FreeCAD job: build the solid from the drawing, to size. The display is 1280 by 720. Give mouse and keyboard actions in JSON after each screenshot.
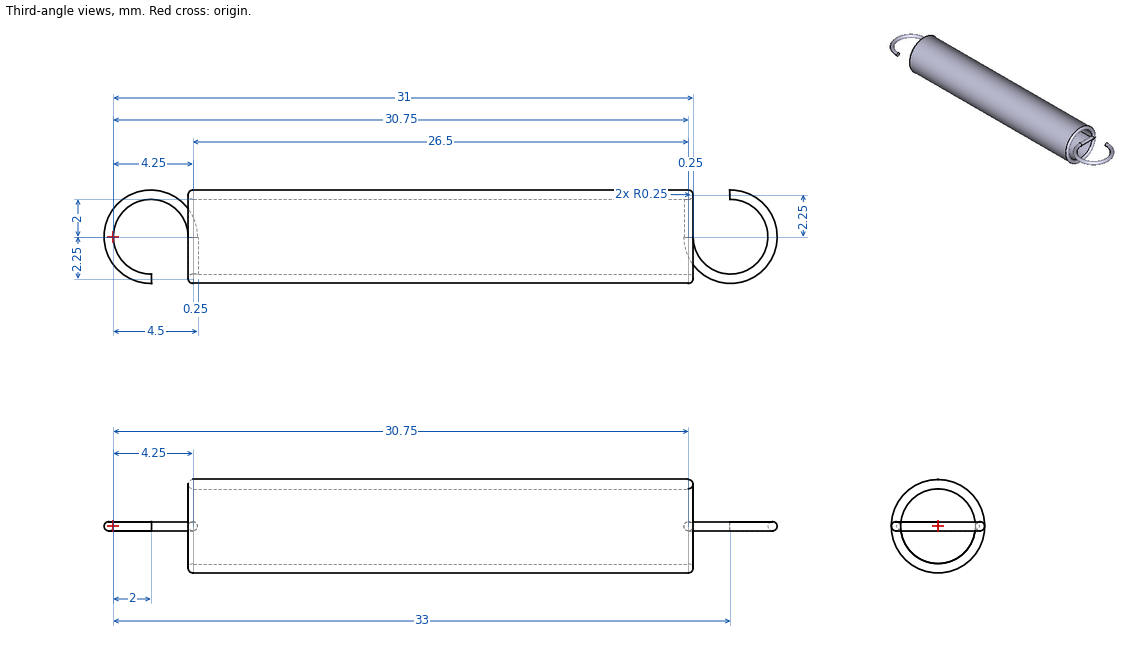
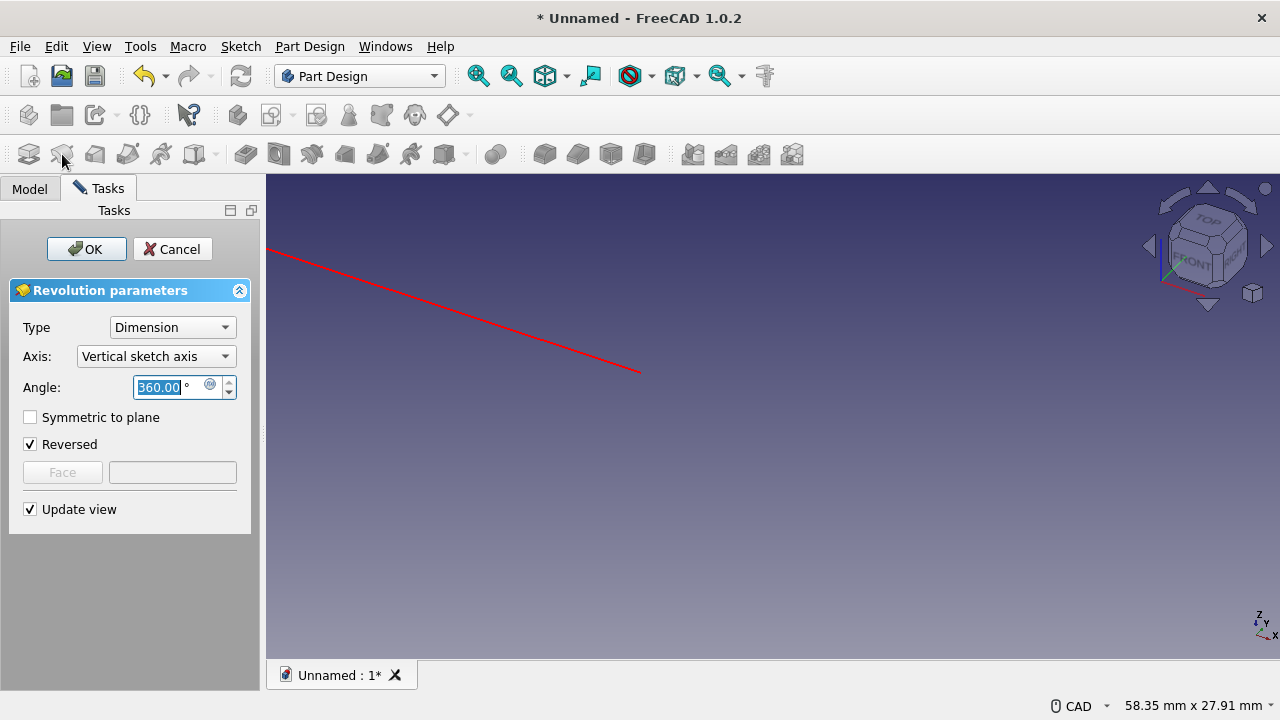
{"action": "left_click", "coordinate": [157, 356]}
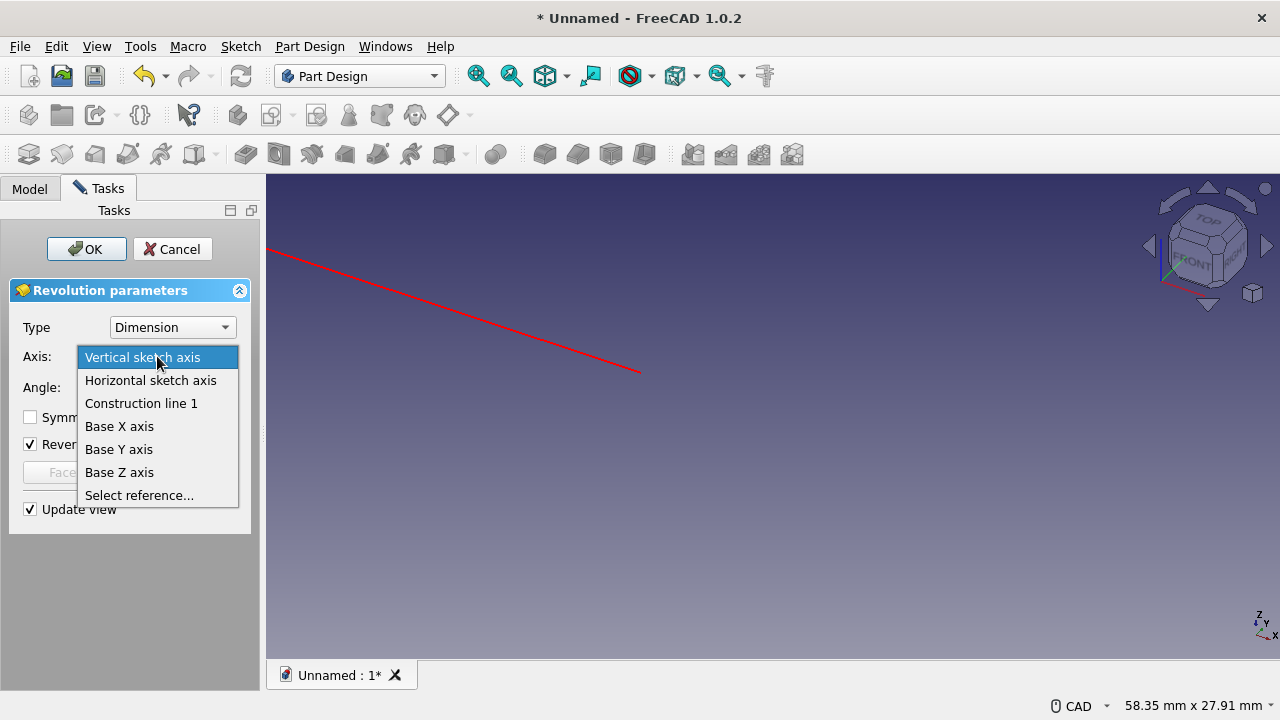
{"action": "left_click", "coordinate": [156, 404]}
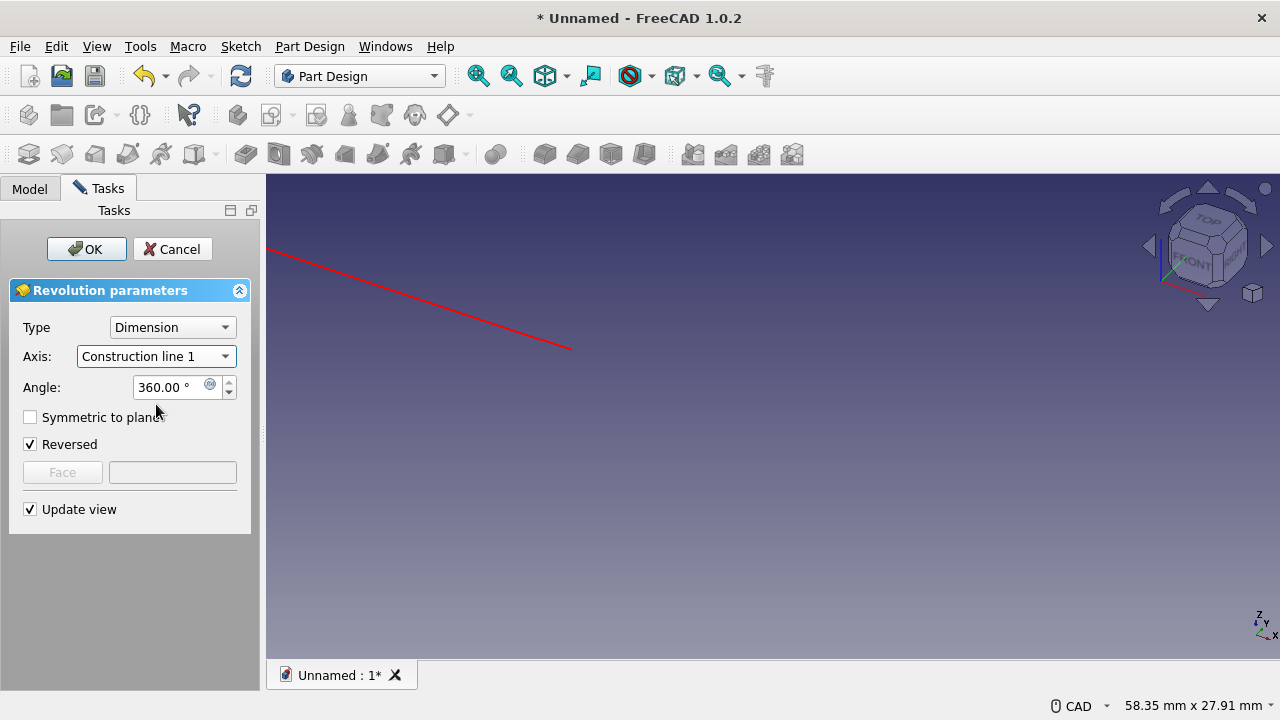
{"action": "left_click", "coordinate": [87, 249]}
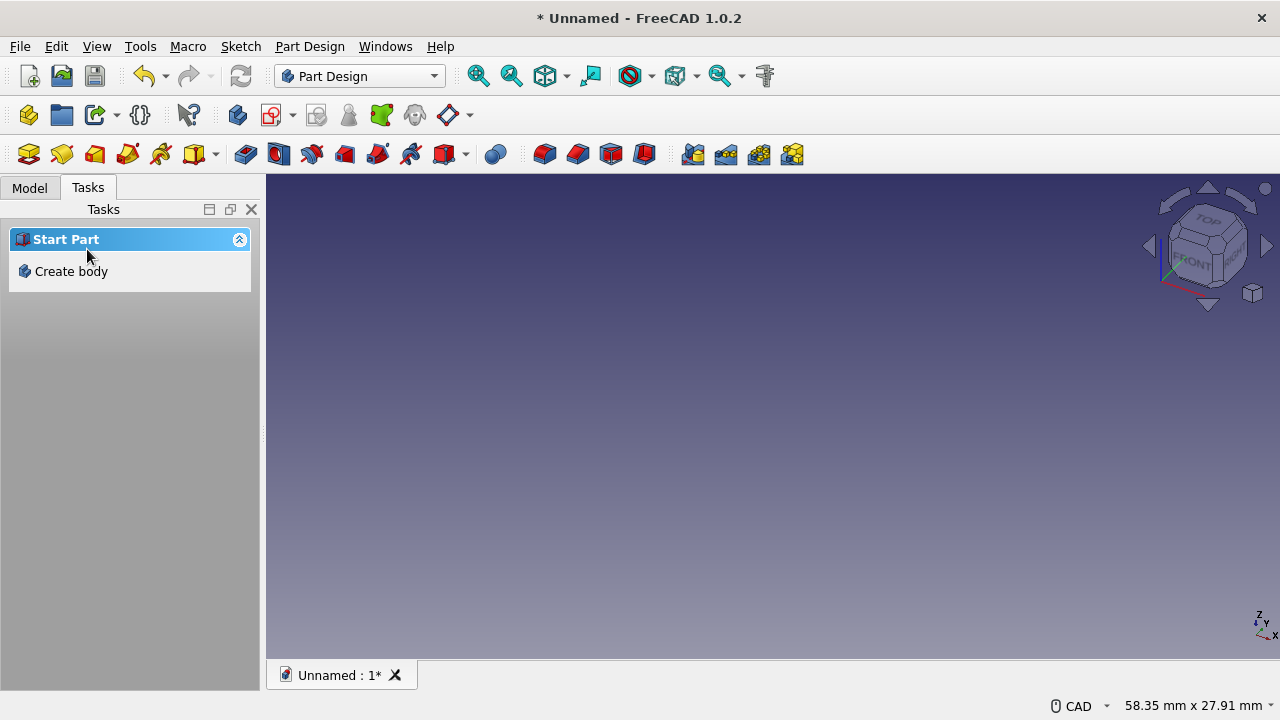
{"action": "key", "text": "v f"}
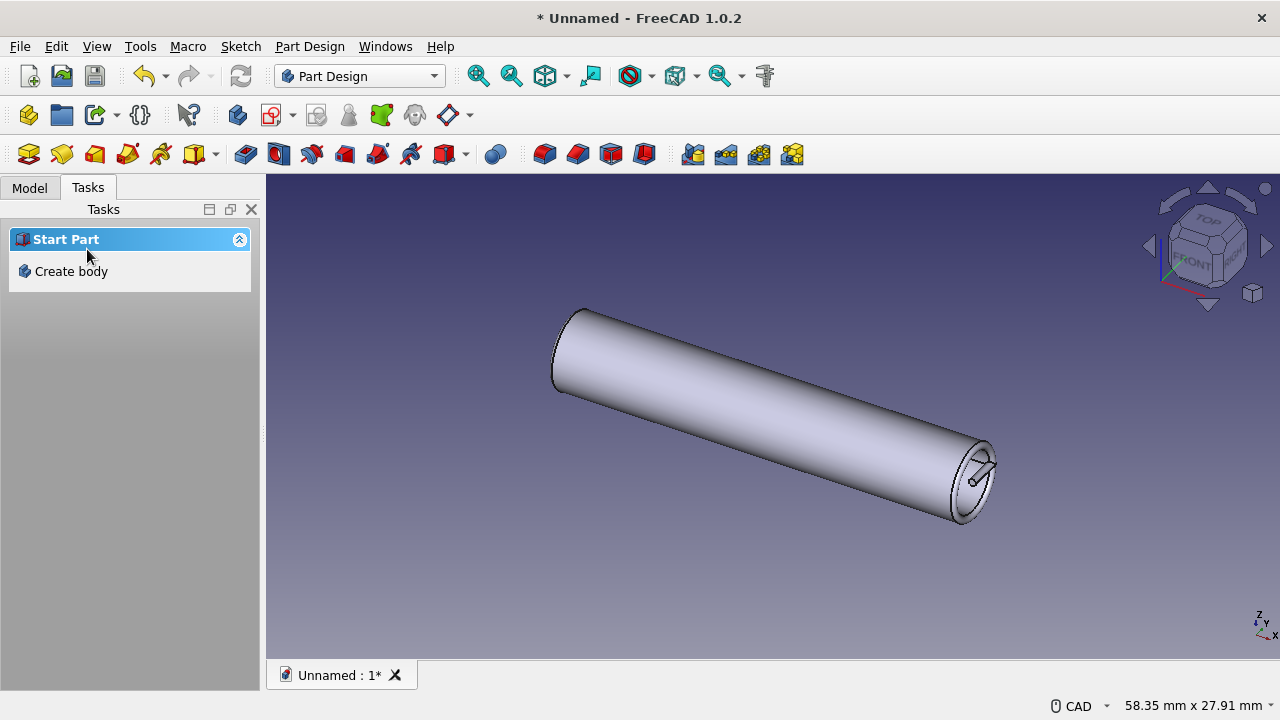
{"action": "left_click", "coordinate": [270, 116]}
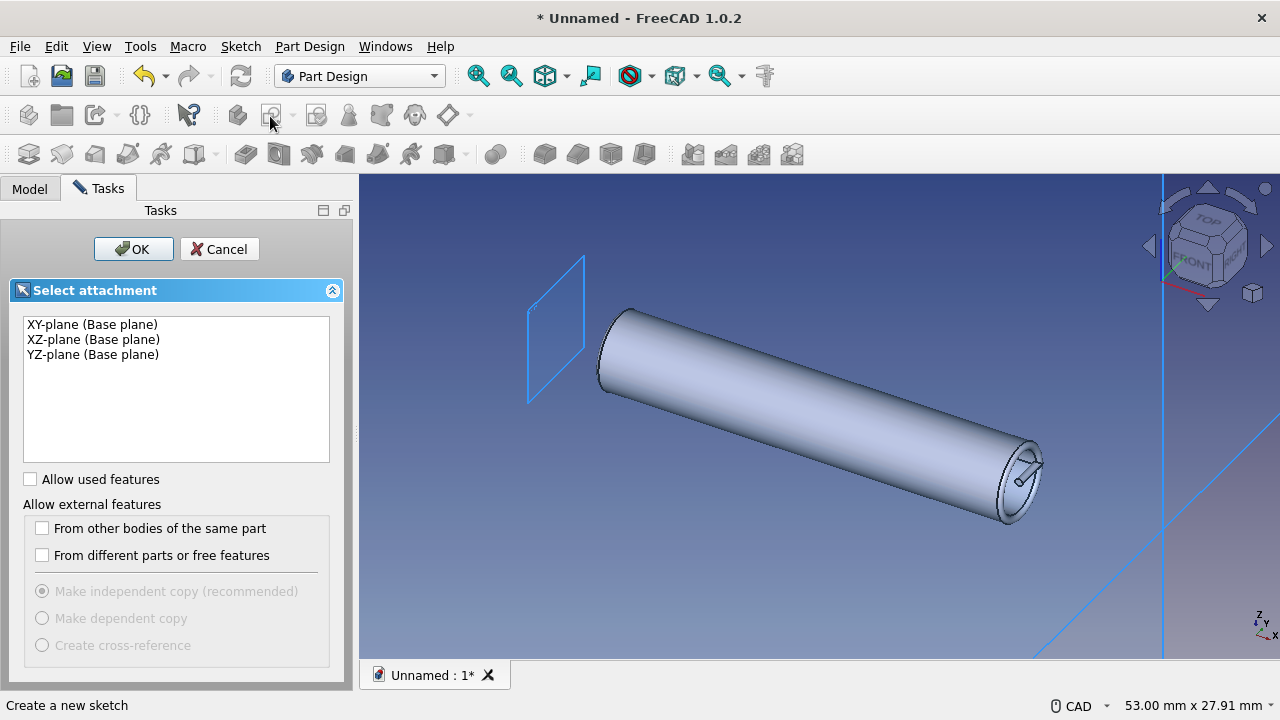
{"action": "left_click", "coordinate": [84, 340]}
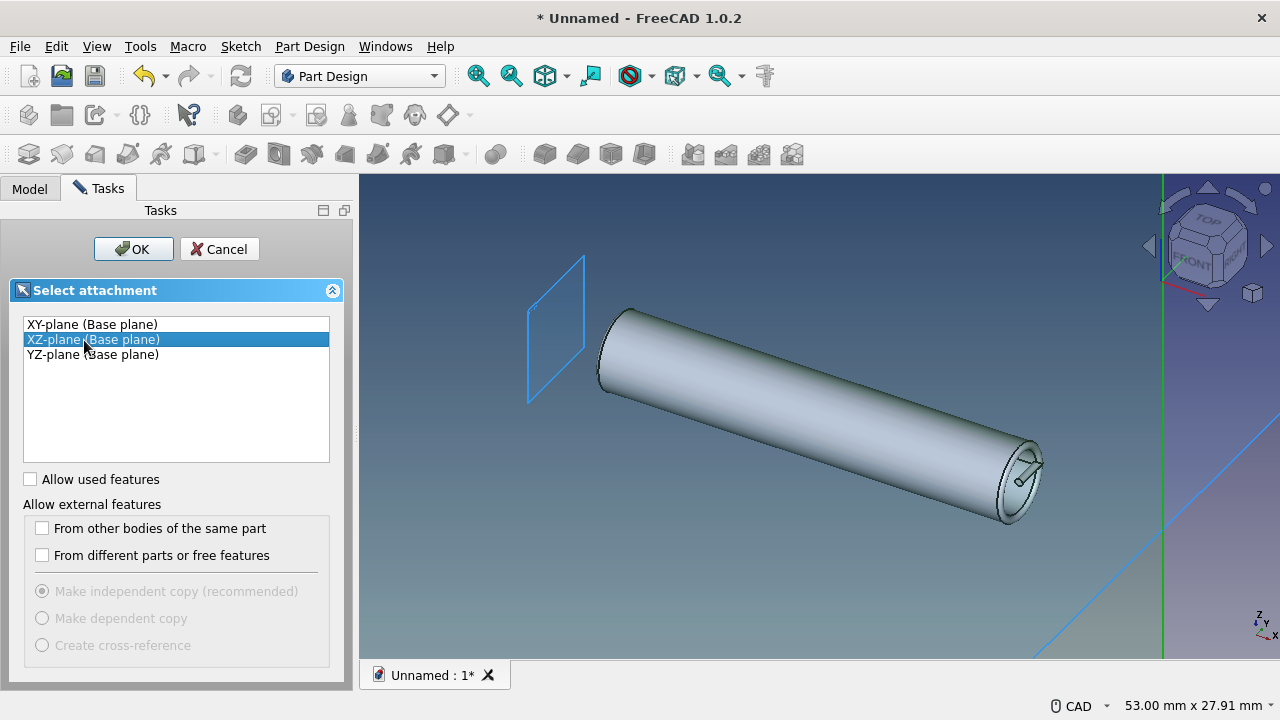
{"action": "left_click", "coordinate": [134, 249]}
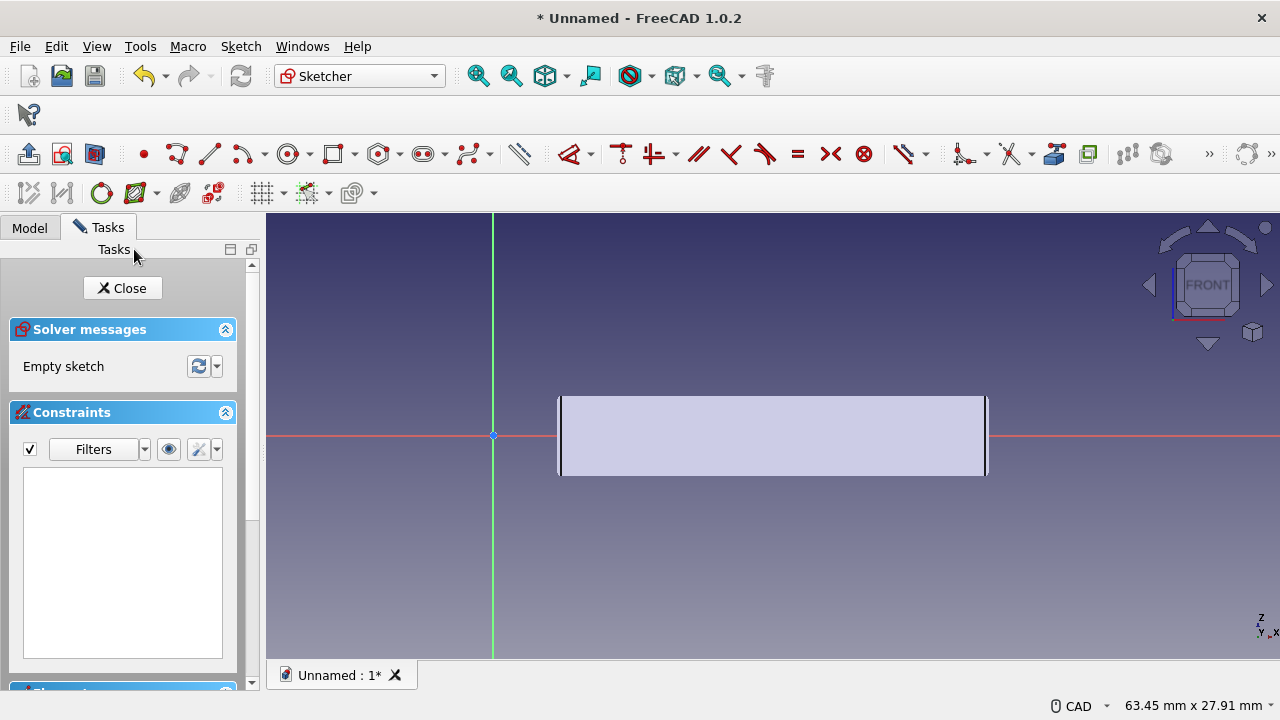
{"action": "key", "text": "q s"}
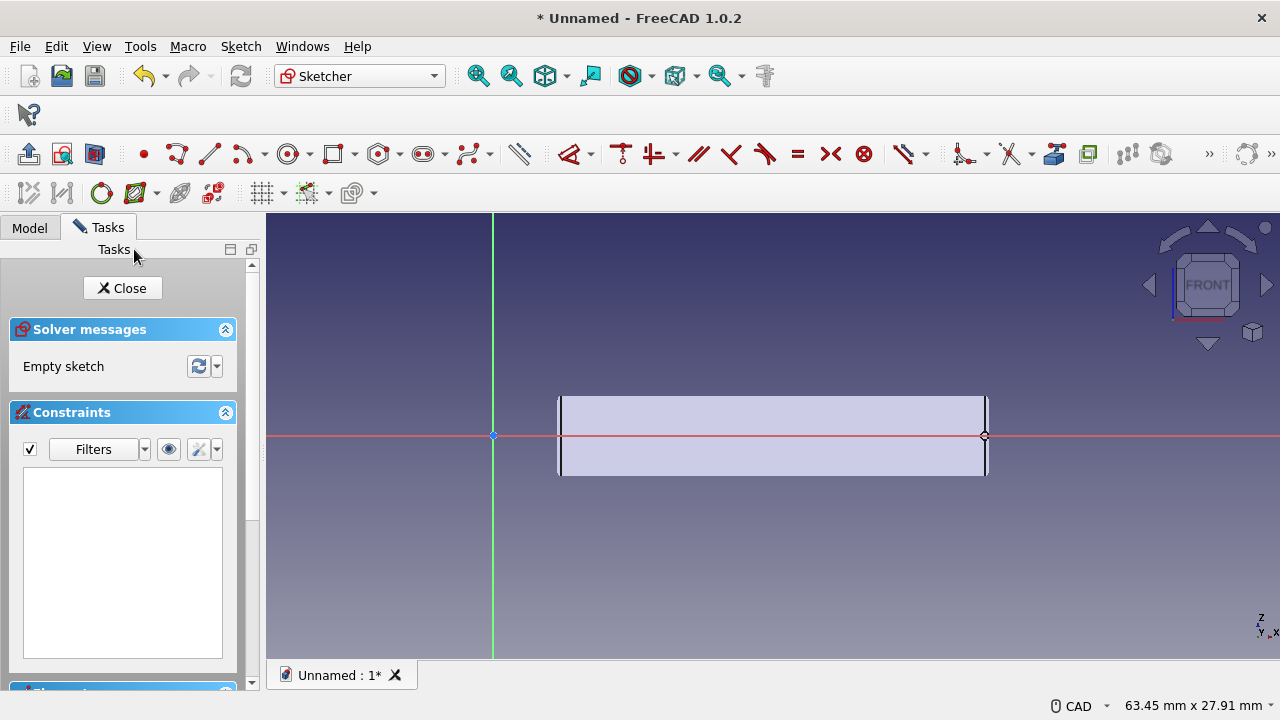
{"action": "scroll", "coordinate": [1024, 436], "scroll_direction": "up", "scroll_amount": 13}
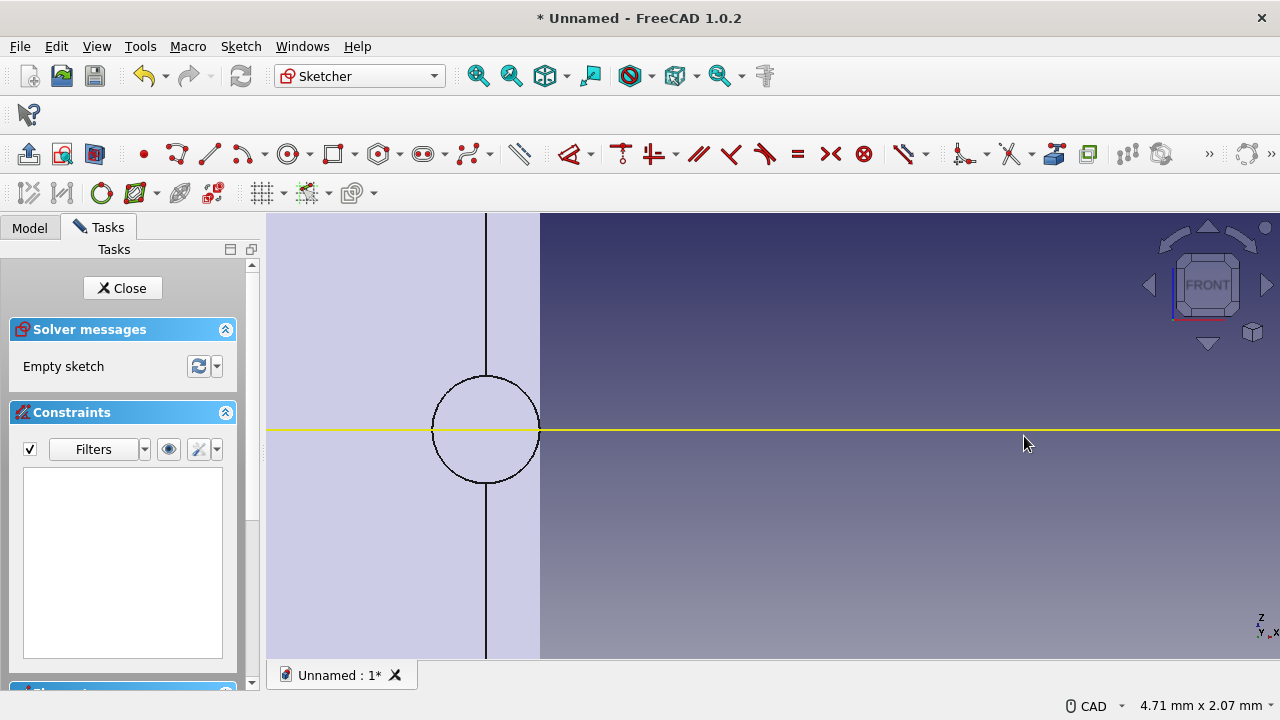
{"action": "key", "text": "g c"}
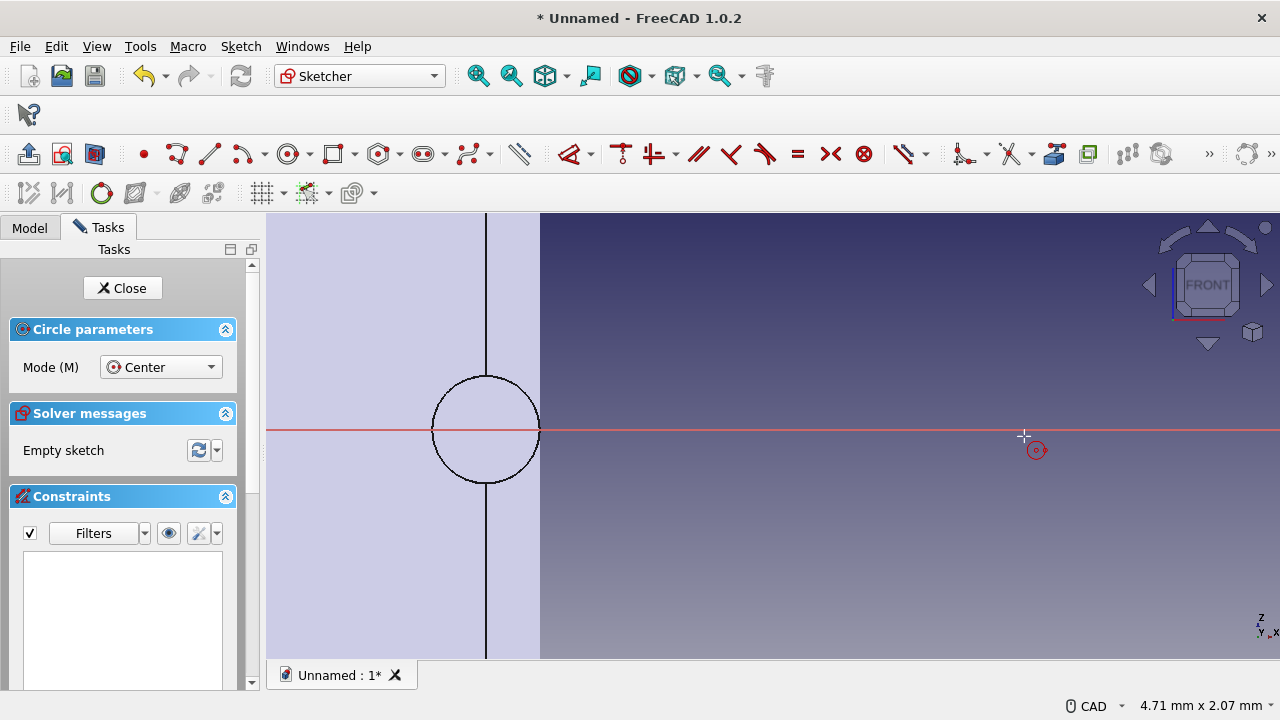
{"action": "left_click", "coordinate": [486, 430]}
{"action": "left_click", "coordinate": [524, 392]}